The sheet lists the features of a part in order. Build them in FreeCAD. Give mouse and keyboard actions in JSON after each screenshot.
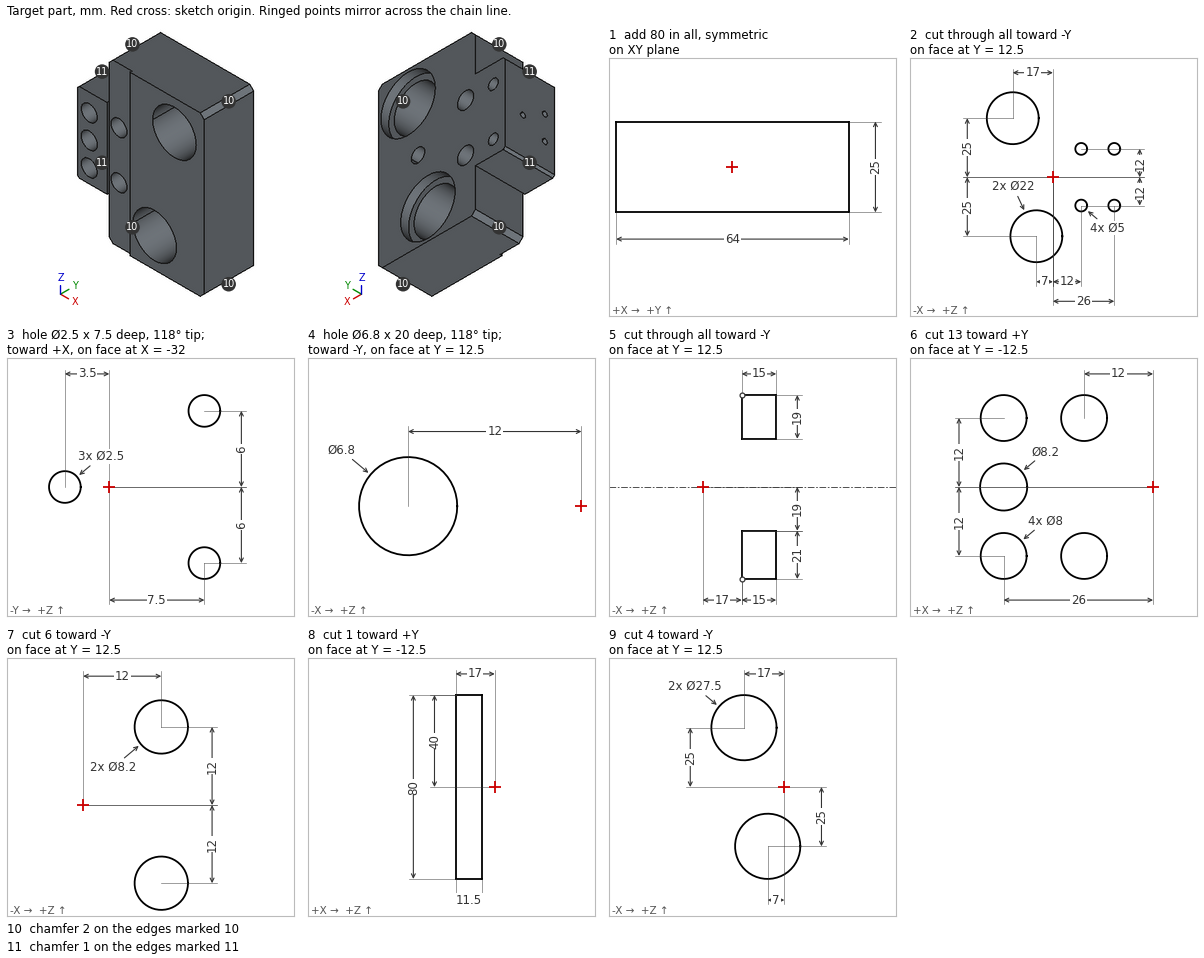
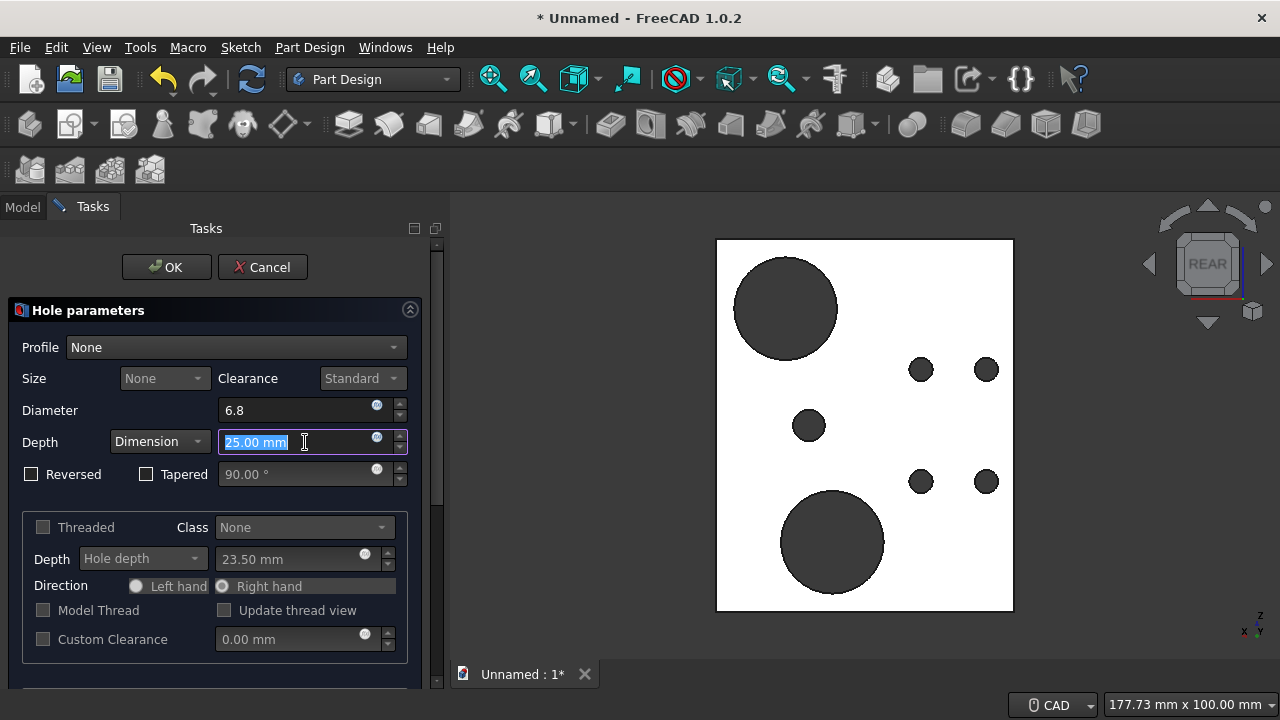
{"action": "type", "text": "20"}
{"action": "key", "text": "Tab"}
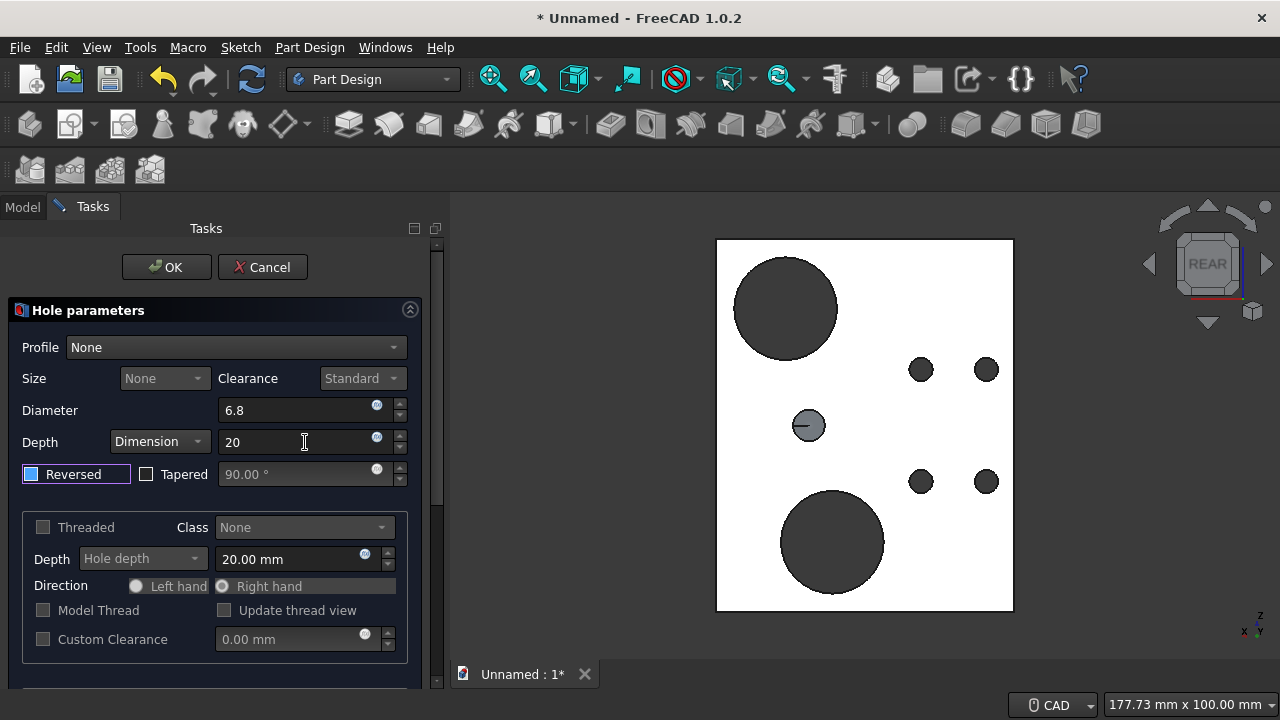
{"action": "left_click", "coordinate": [167, 267]}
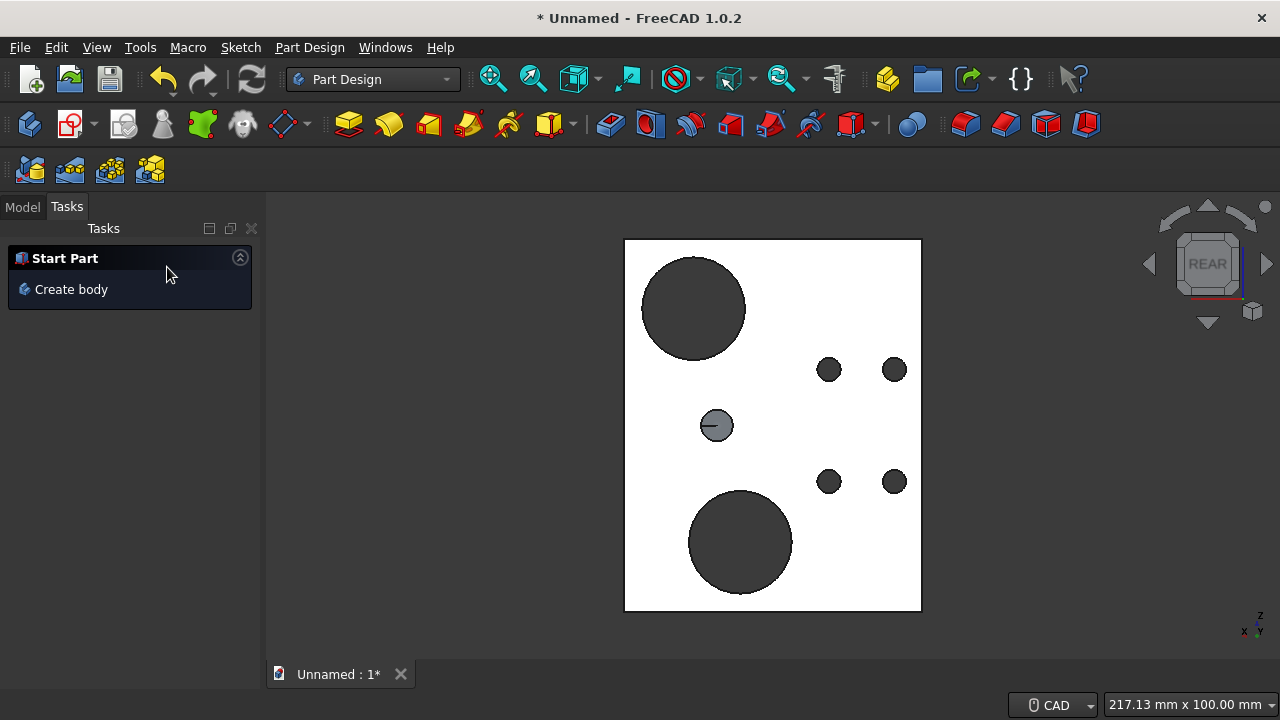
{"action": "left_click", "coordinate": [858, 425]}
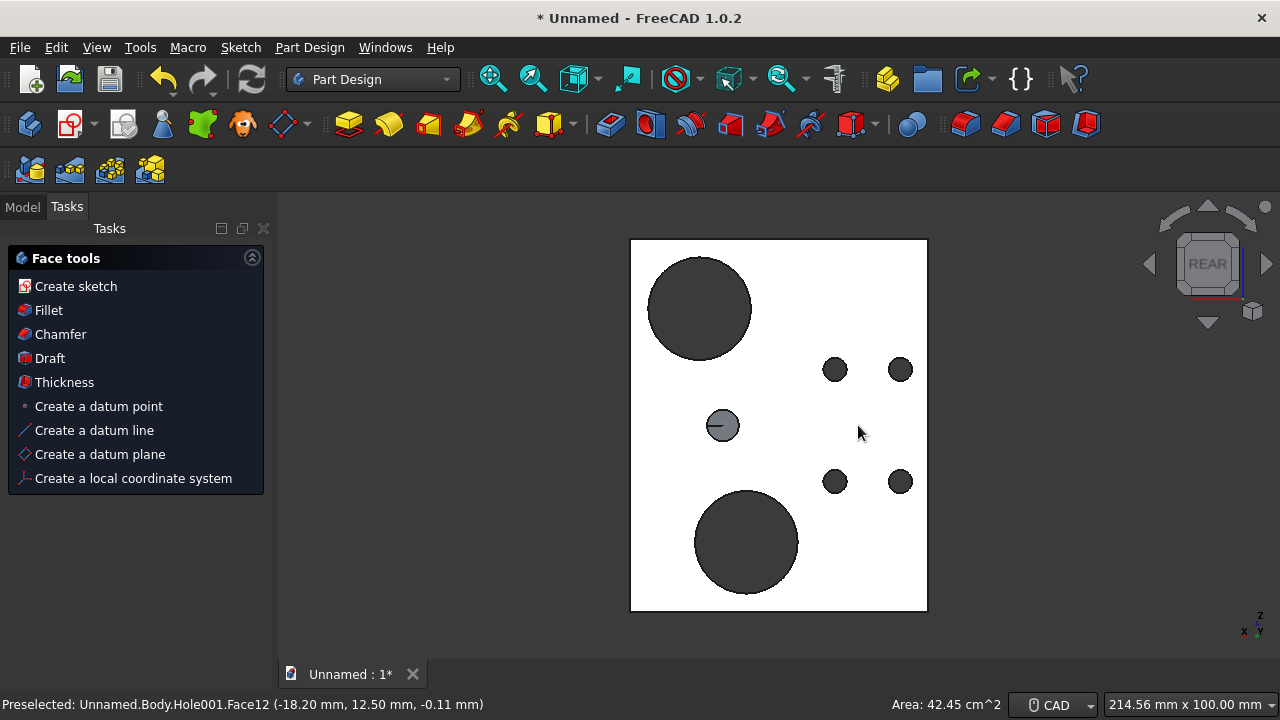
{"action": "left_click", "coordinate": [70, 124]}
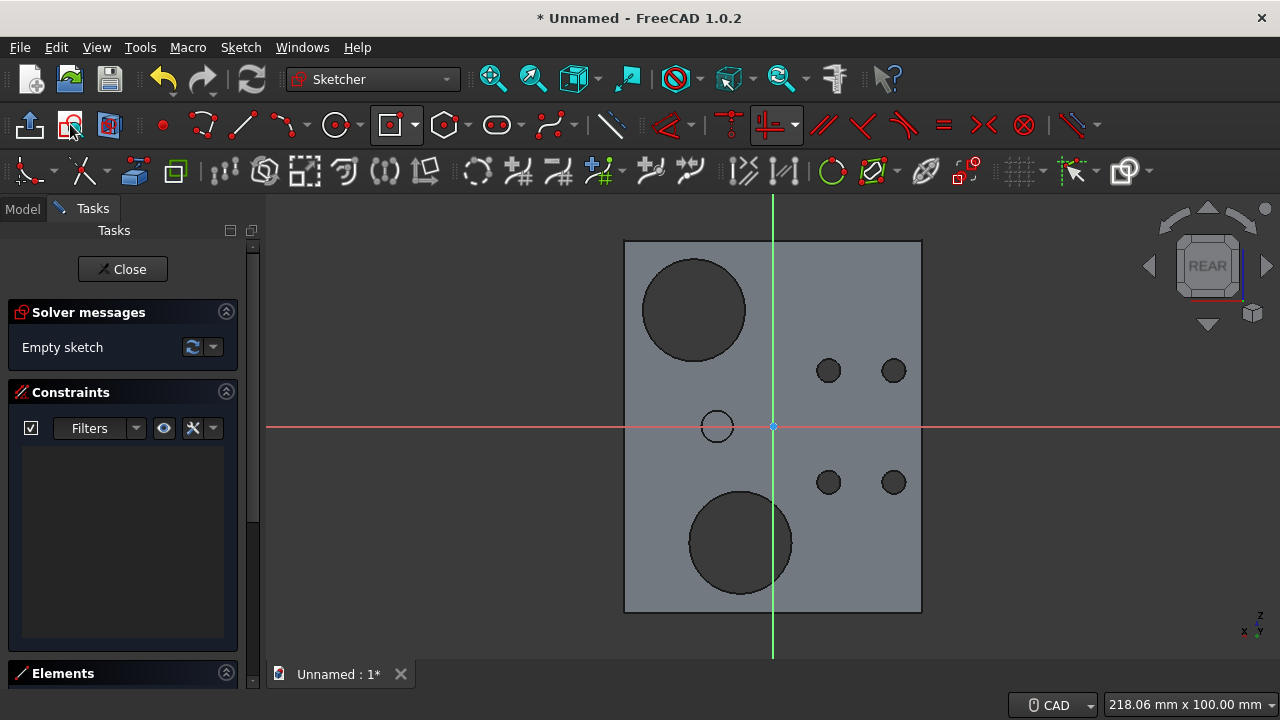
{"action": "scroll", "coordinate": [294, 426], "scroll_direction": "down", "scroll_amount": 1}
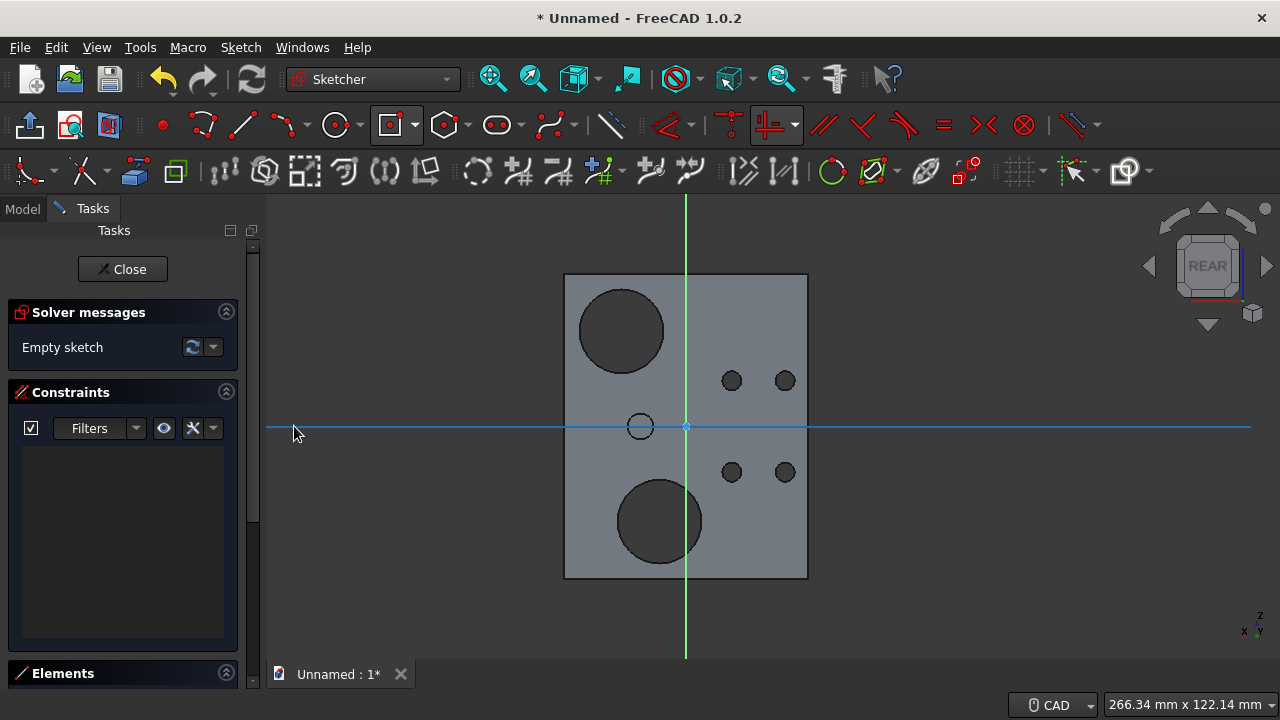
{"action": "left_click", "coordinate": [418, 126]}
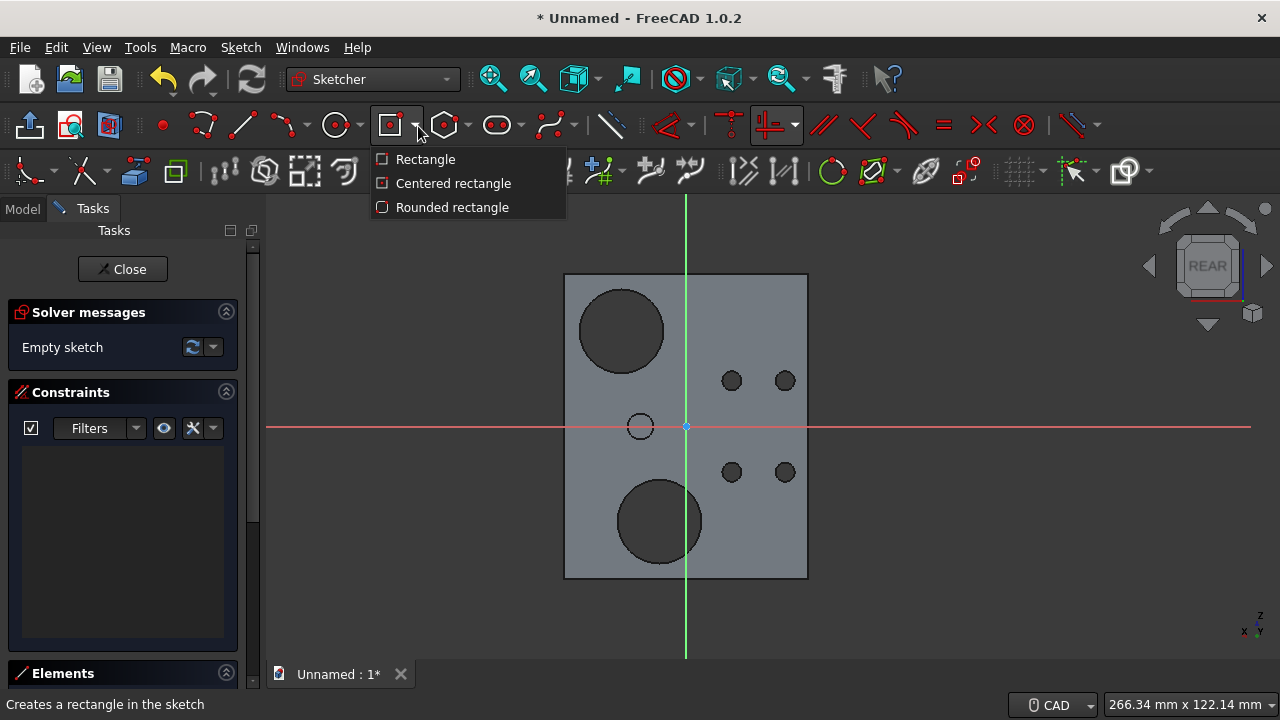
{"action": "left_click", "coordinate": [468, 159]}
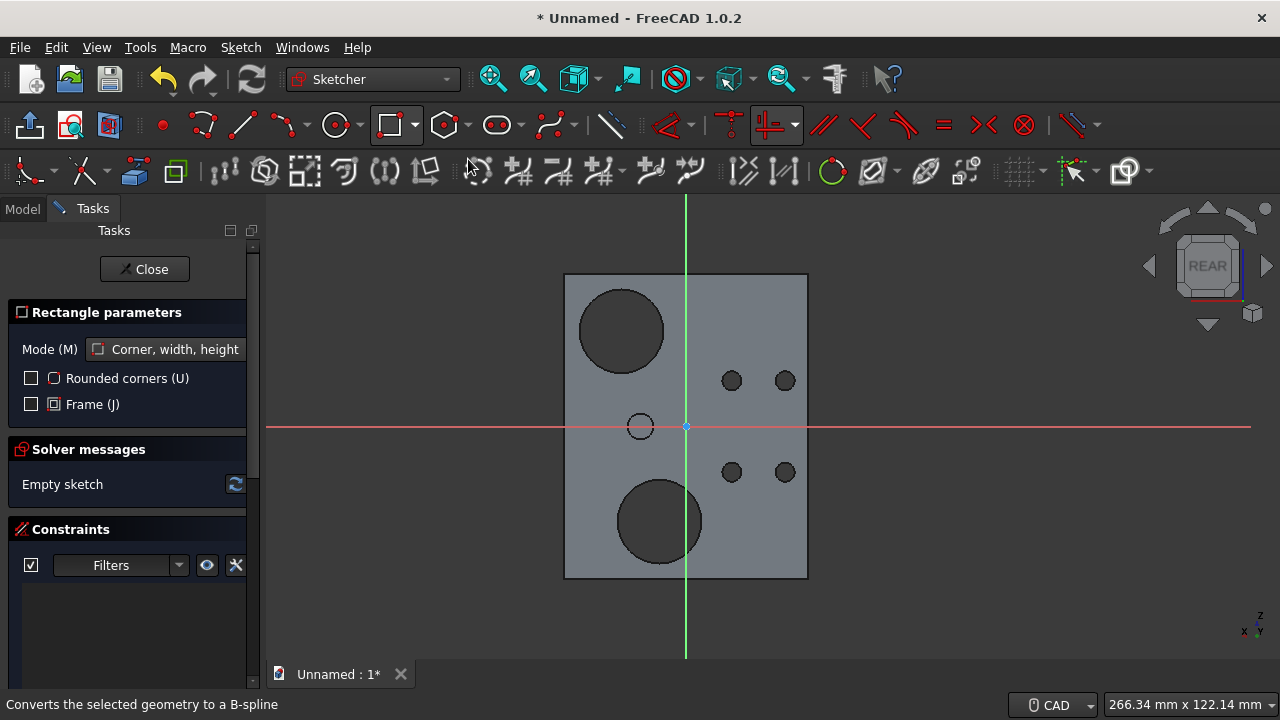
{"action": "left_click", "coordinate": [751, 499]}
{"action": "left_click", "coordinate": [808, 579]}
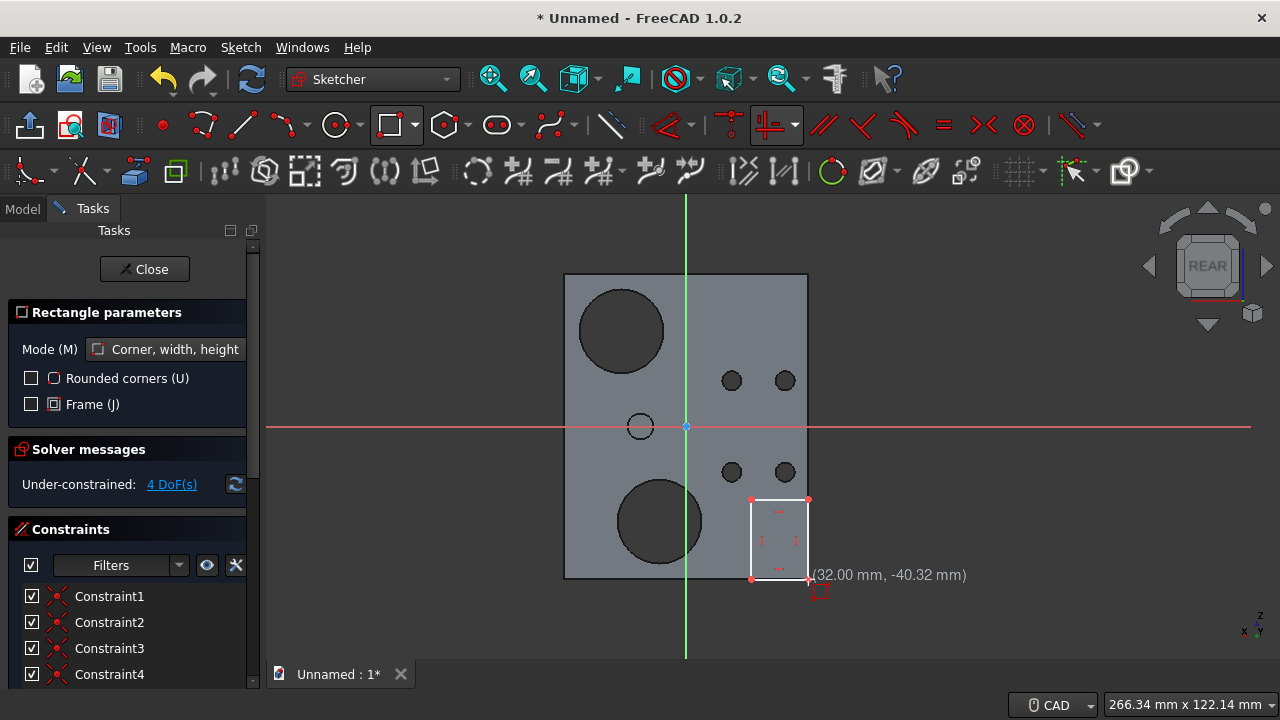
{"action": "left_click", "coordinate": [751, 274]}
{"action": "left_click", "coordinate": [808, 347]}
{"action": "key", "text": "Escape"}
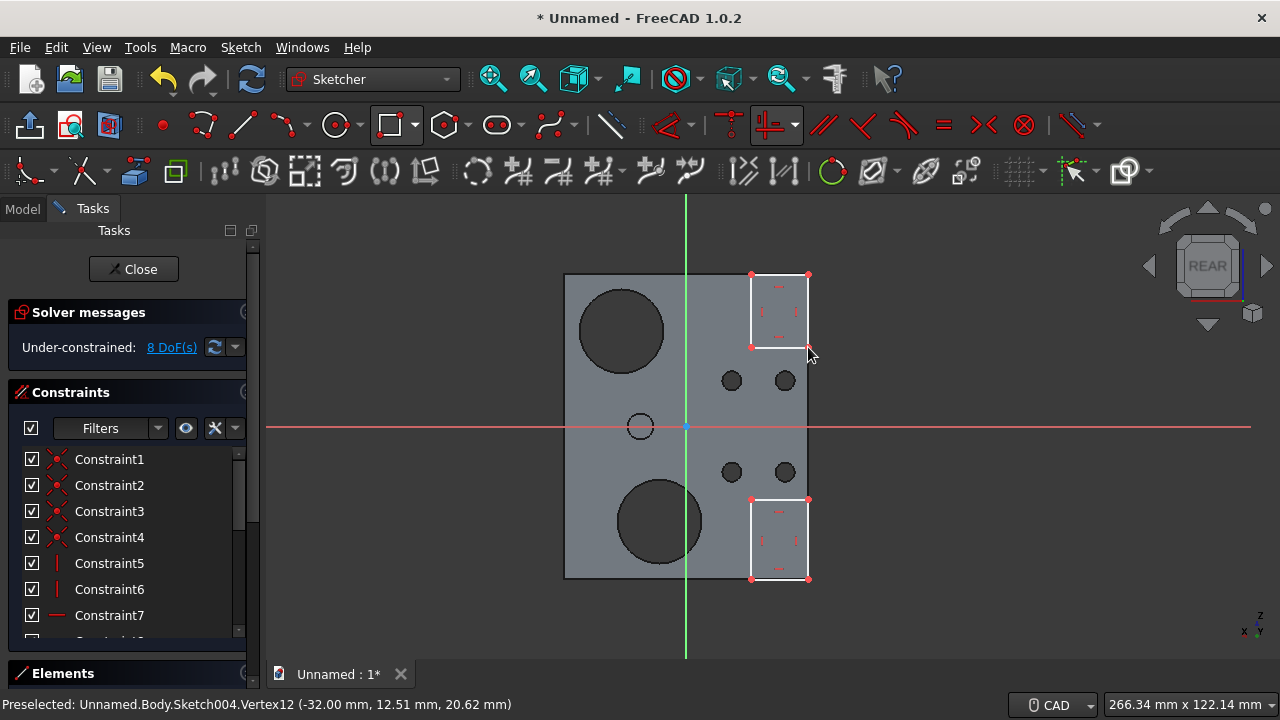
{"action": "left_click", "coordinate": [751, 580]}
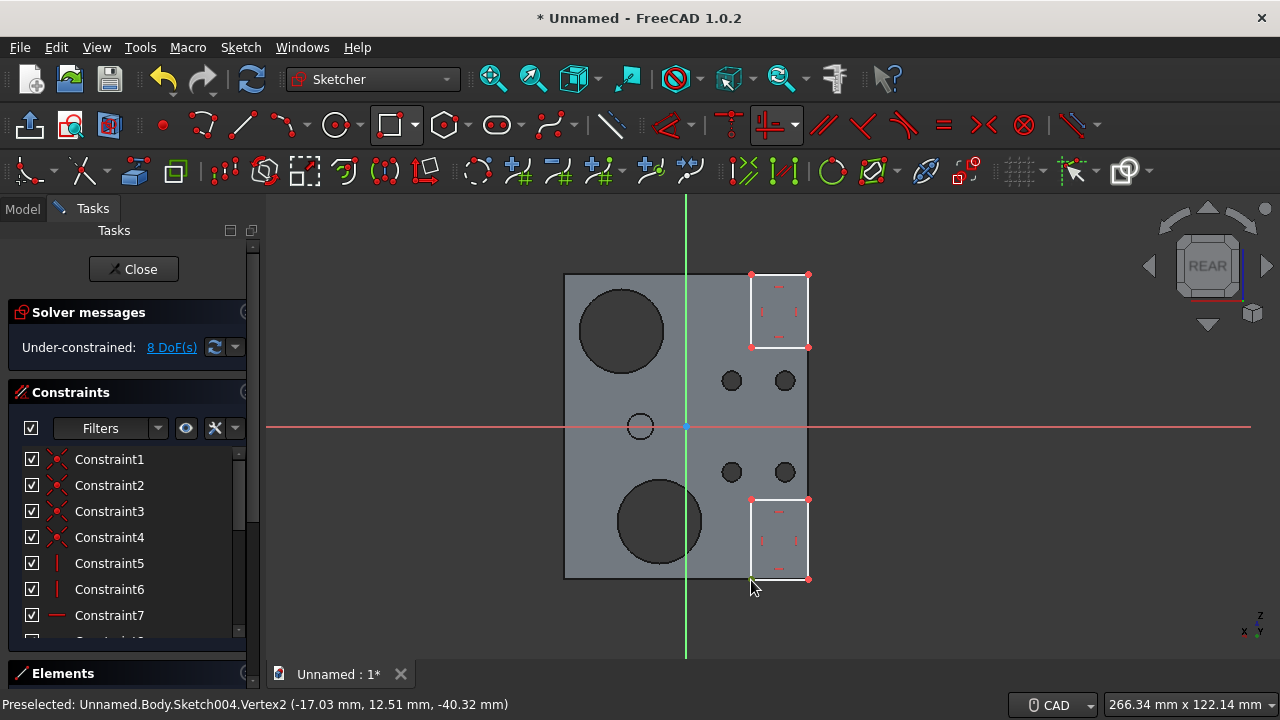
{"action": "left_click", "coordinate": [751, 275]}